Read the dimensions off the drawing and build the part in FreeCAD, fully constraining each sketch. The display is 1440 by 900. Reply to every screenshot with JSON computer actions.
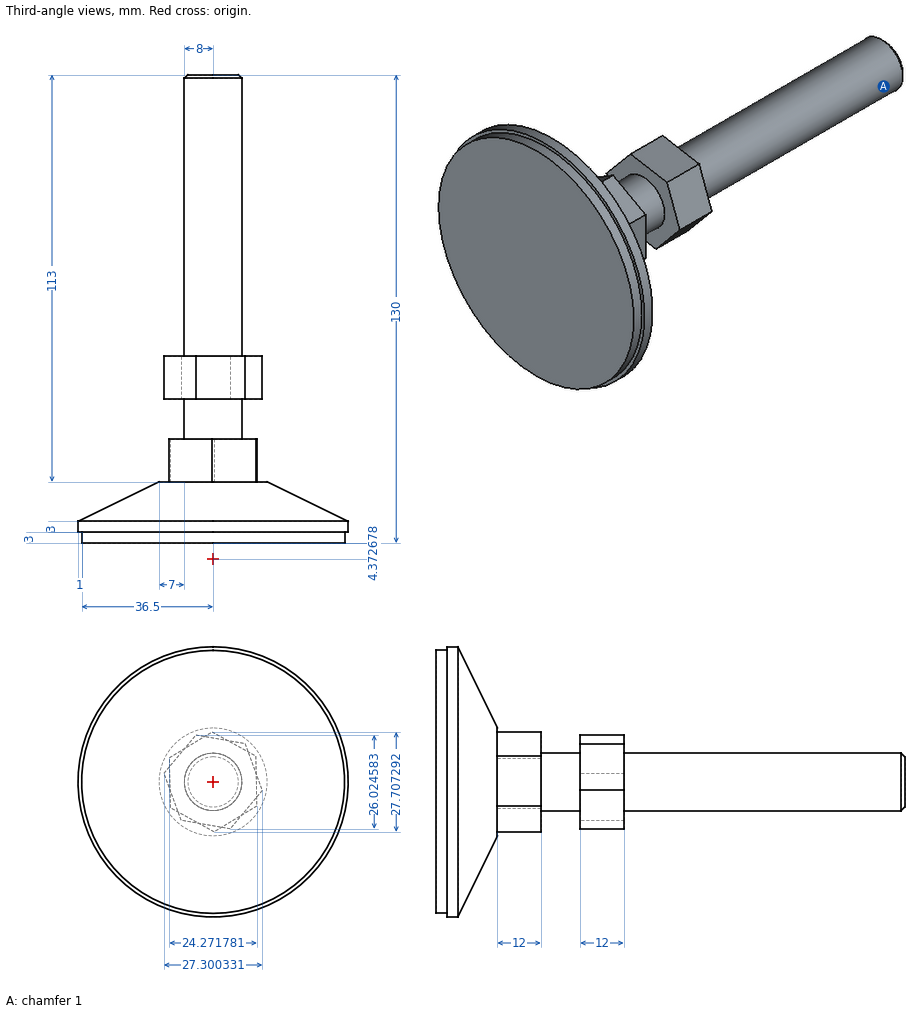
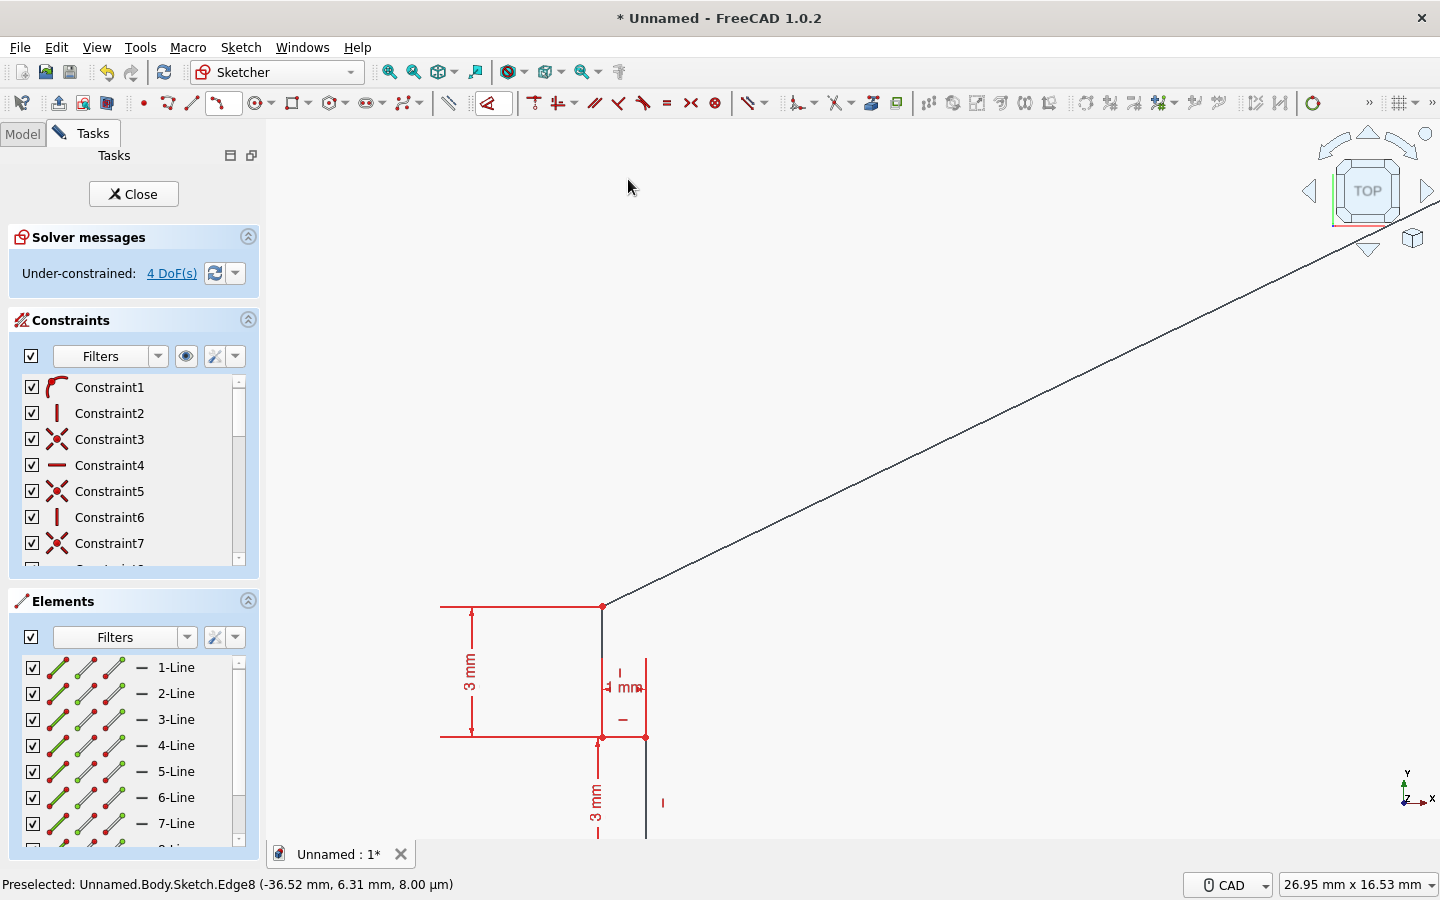
{"action": "scroll", "coordinate": [734, 668], "scroll_direction": "down", "scroll_amount": 13}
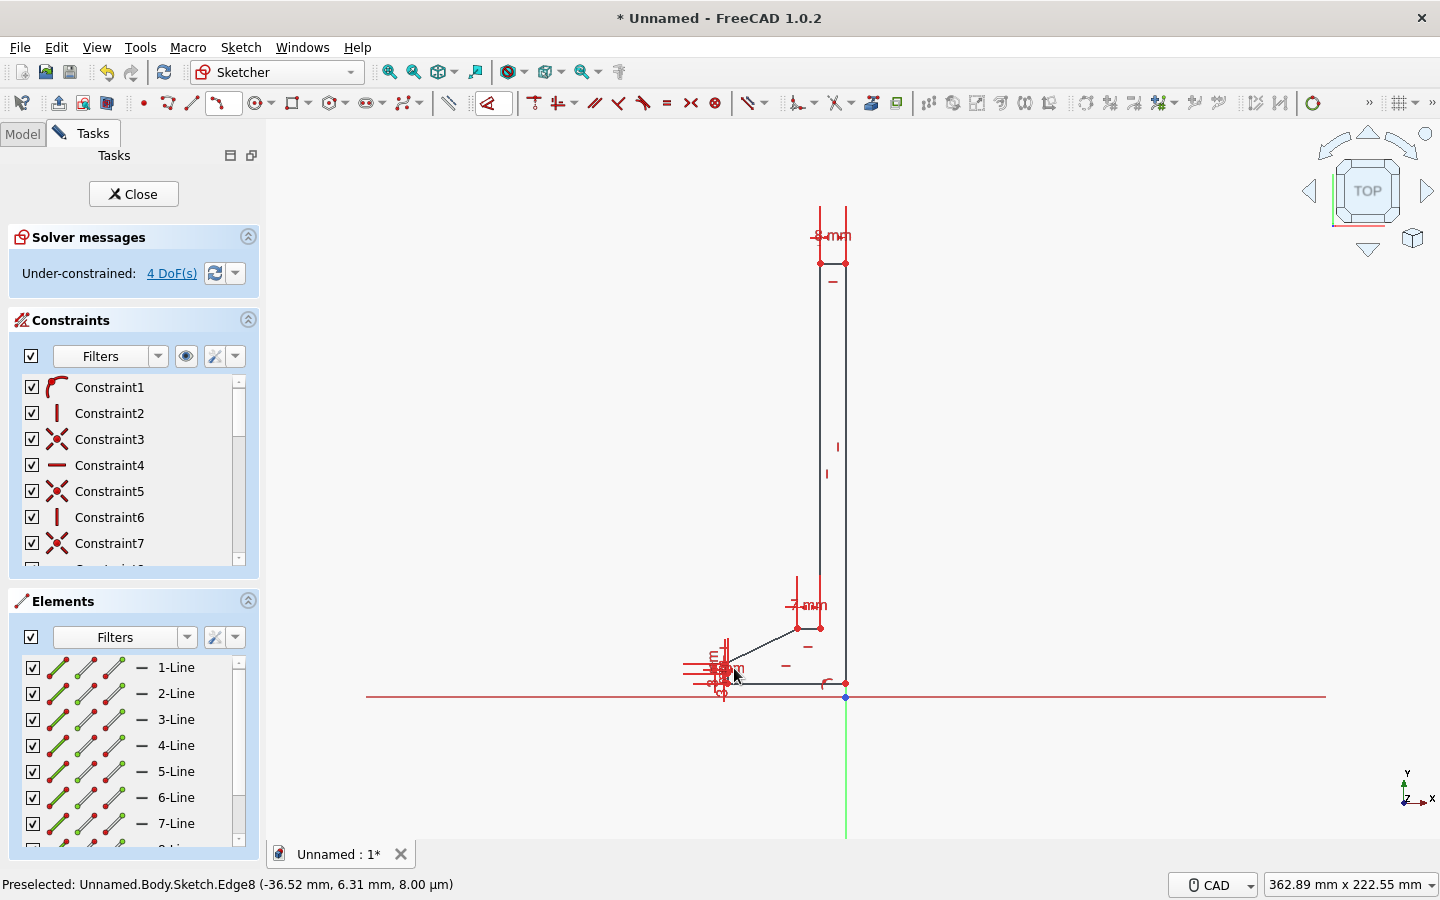
{"action": "left_click", "coordinate": [846, 558]}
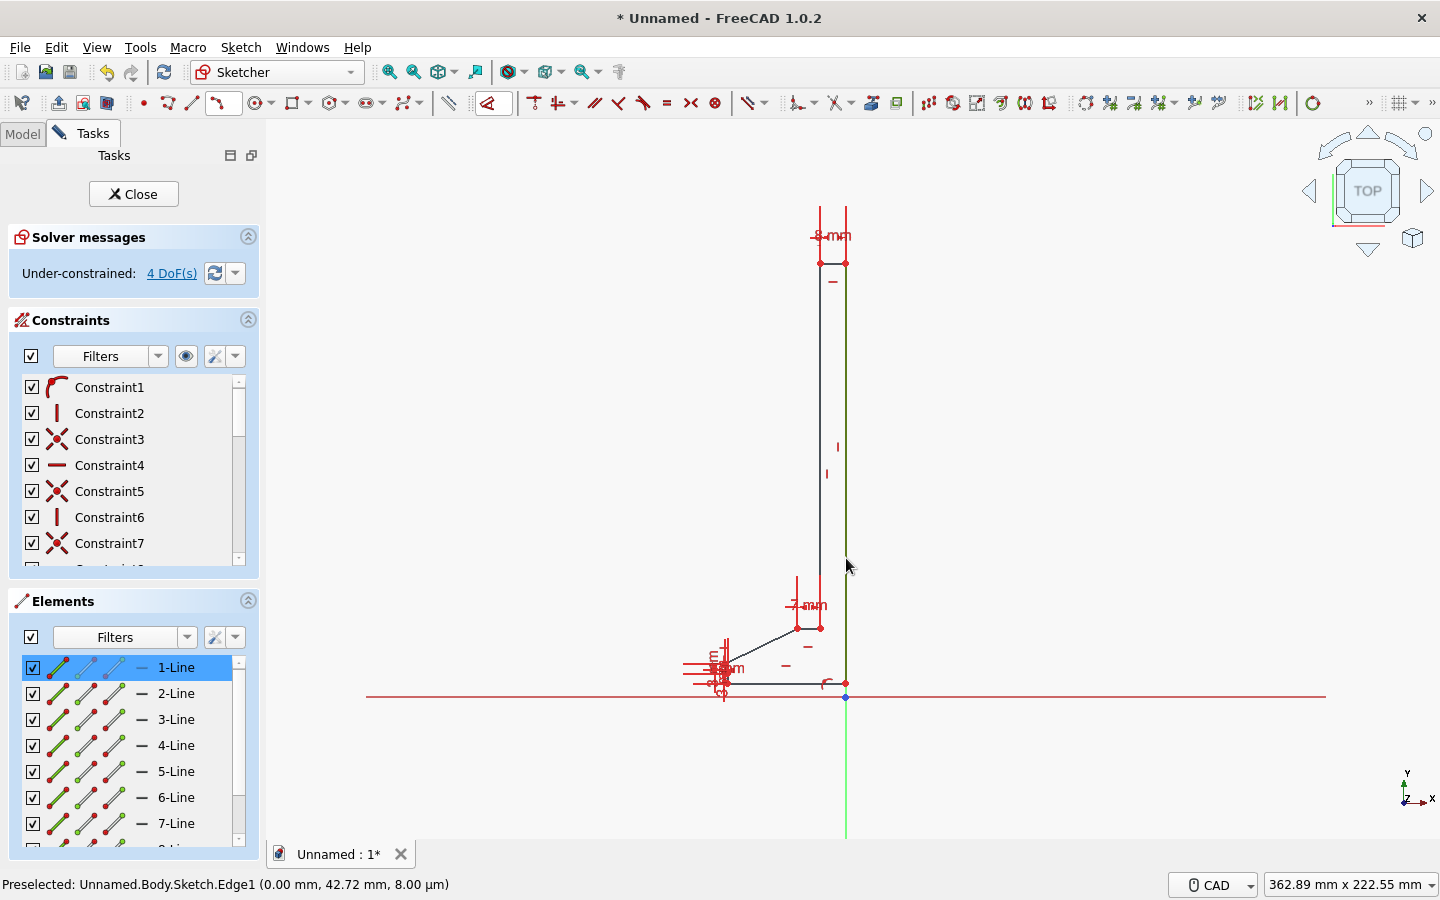
{"action": "key", "text": "i"}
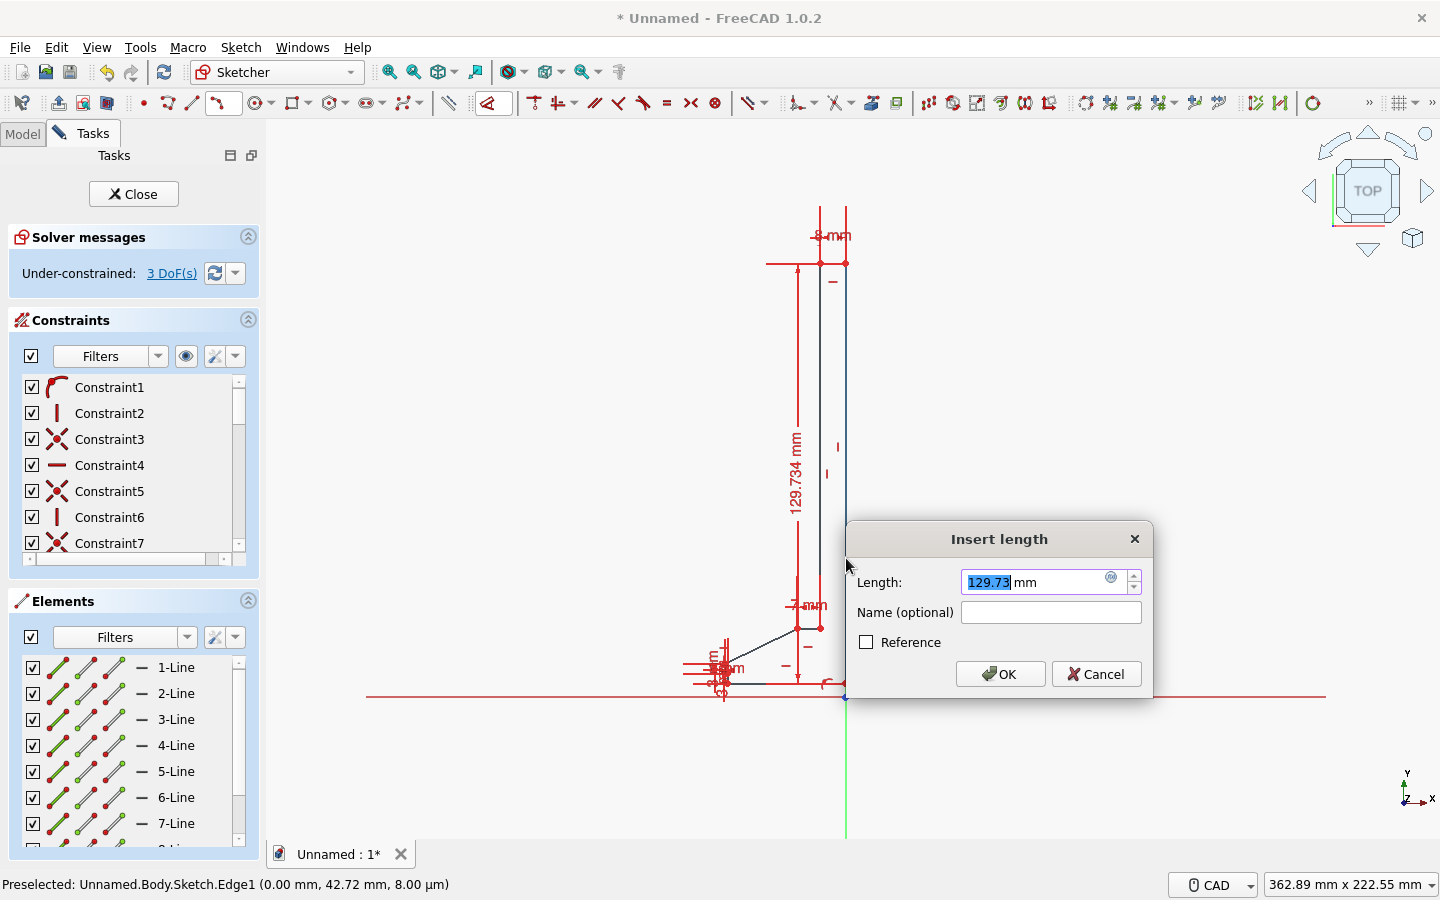
{"action": "type", "text": "130"}
{"action": "key", "text": "Return"}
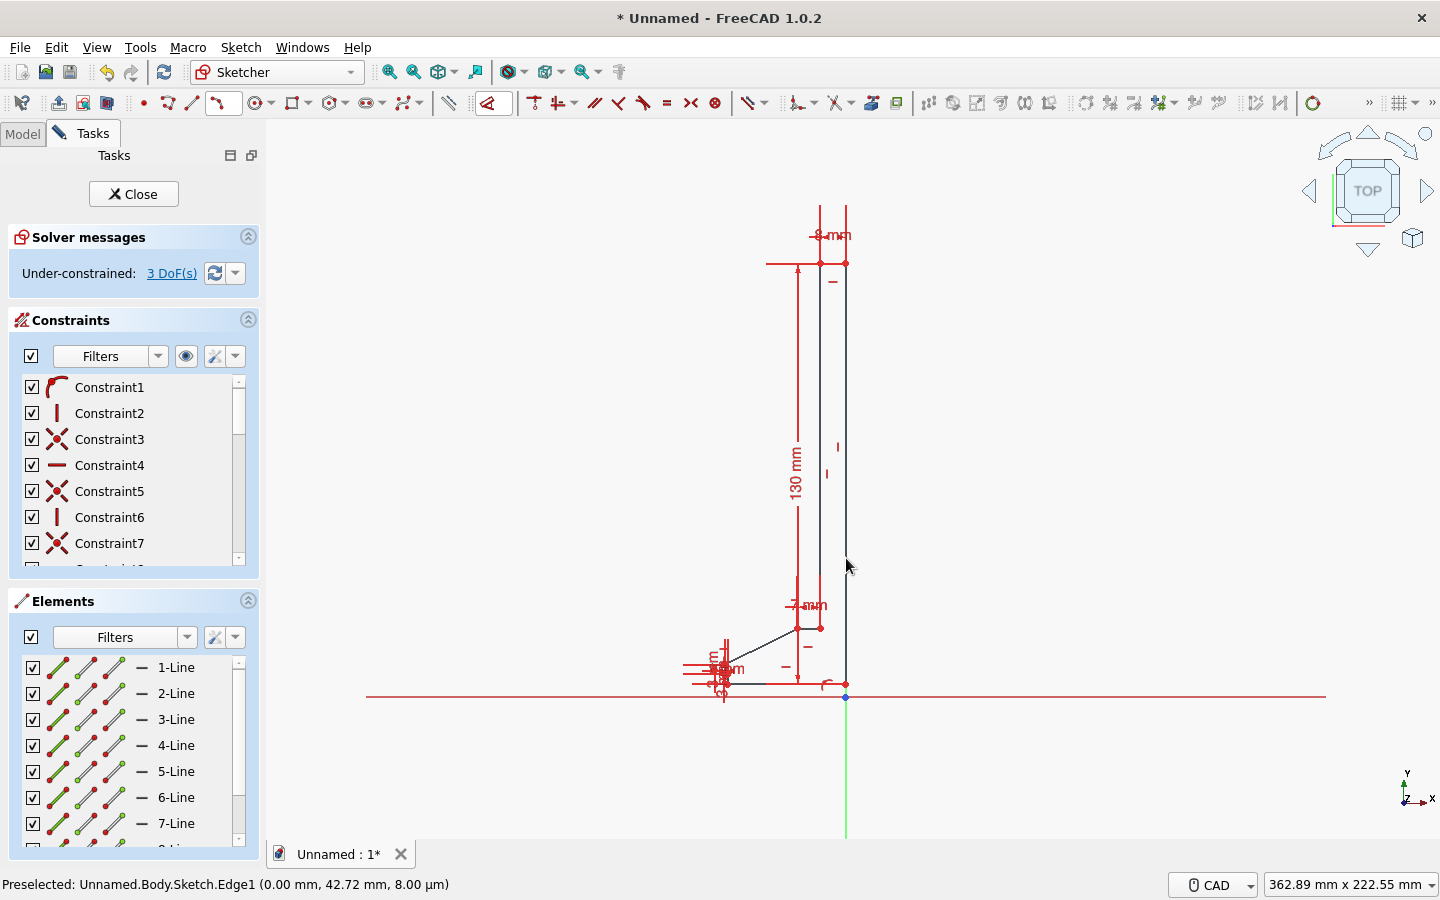
{"action": "left_click", "coordinate": [820, 373]}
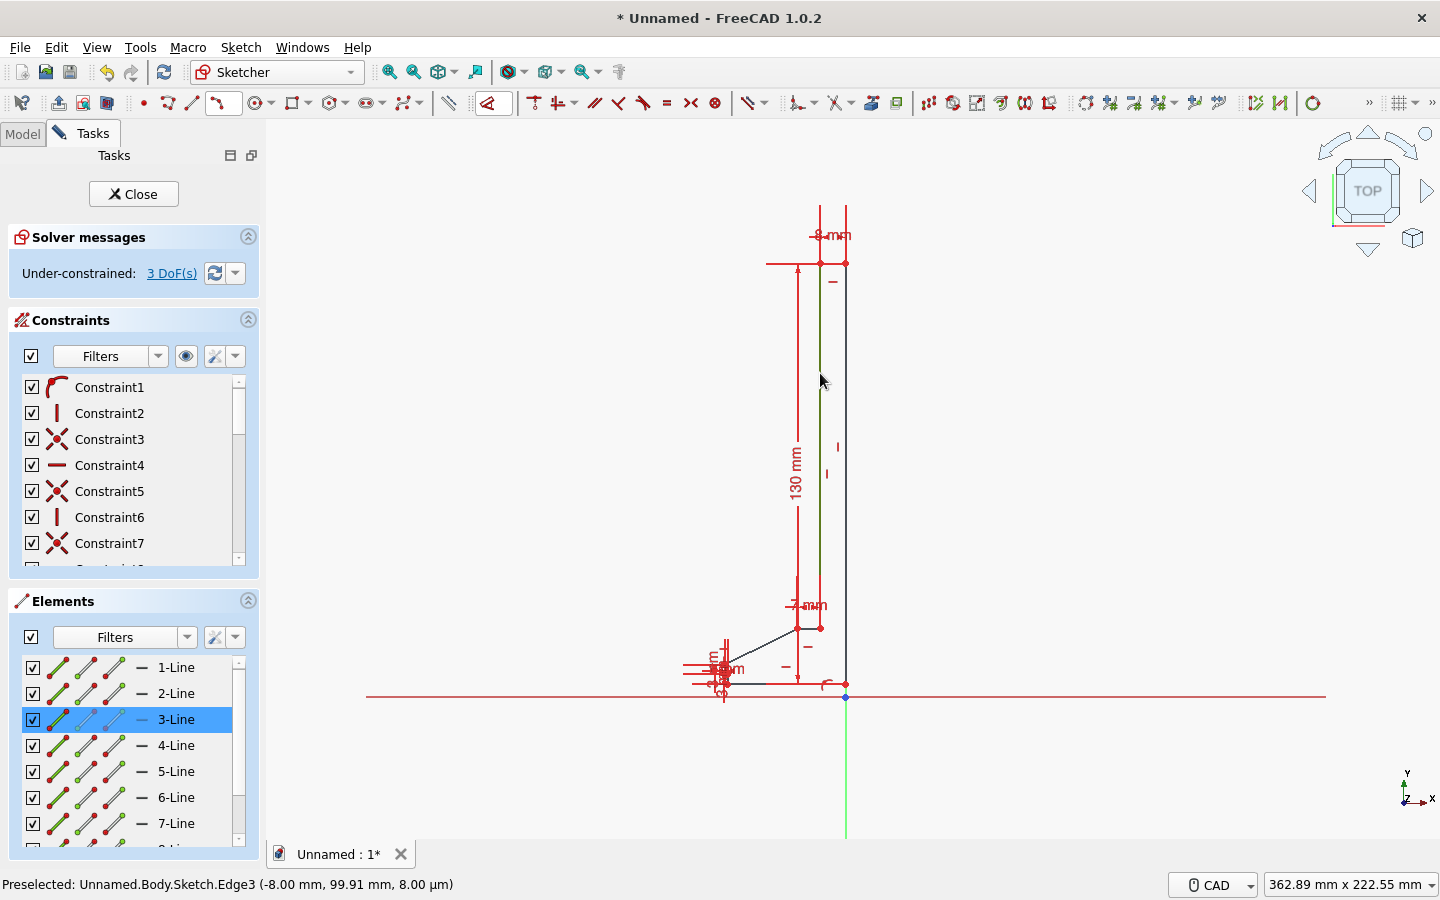
{"action": "left_click", "coordinate": [506, 104]}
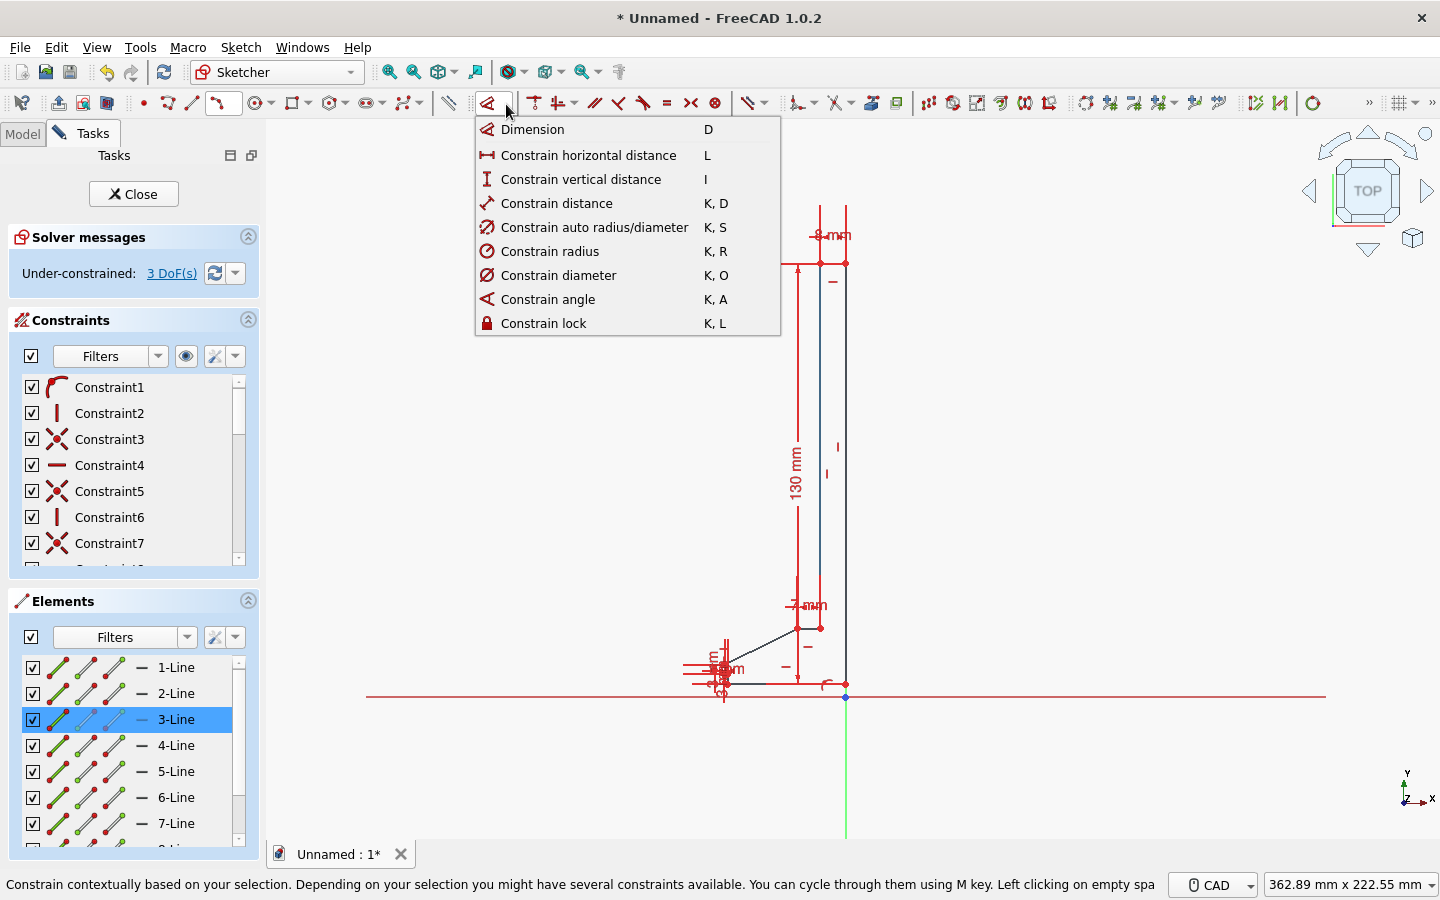
{"action": "left_click", "coordinate": [628, 179]}